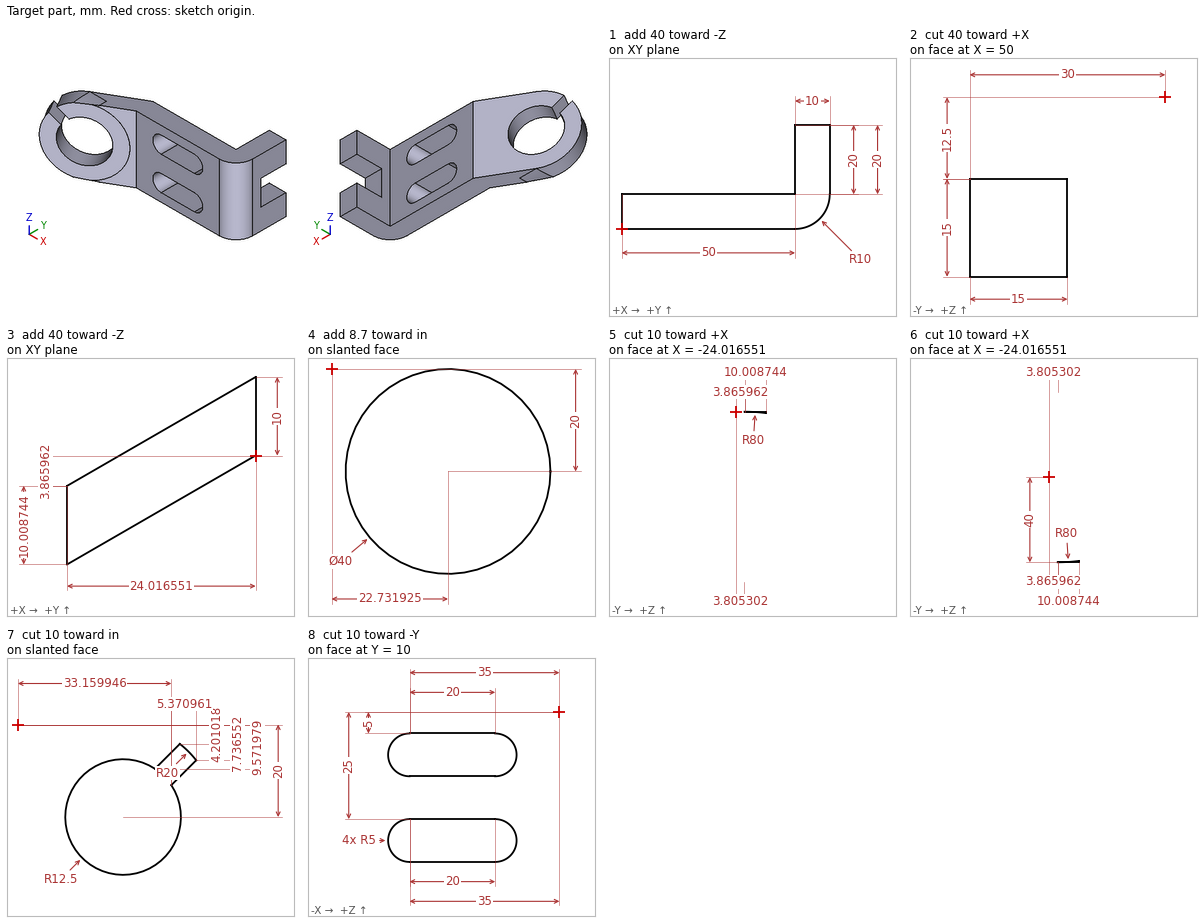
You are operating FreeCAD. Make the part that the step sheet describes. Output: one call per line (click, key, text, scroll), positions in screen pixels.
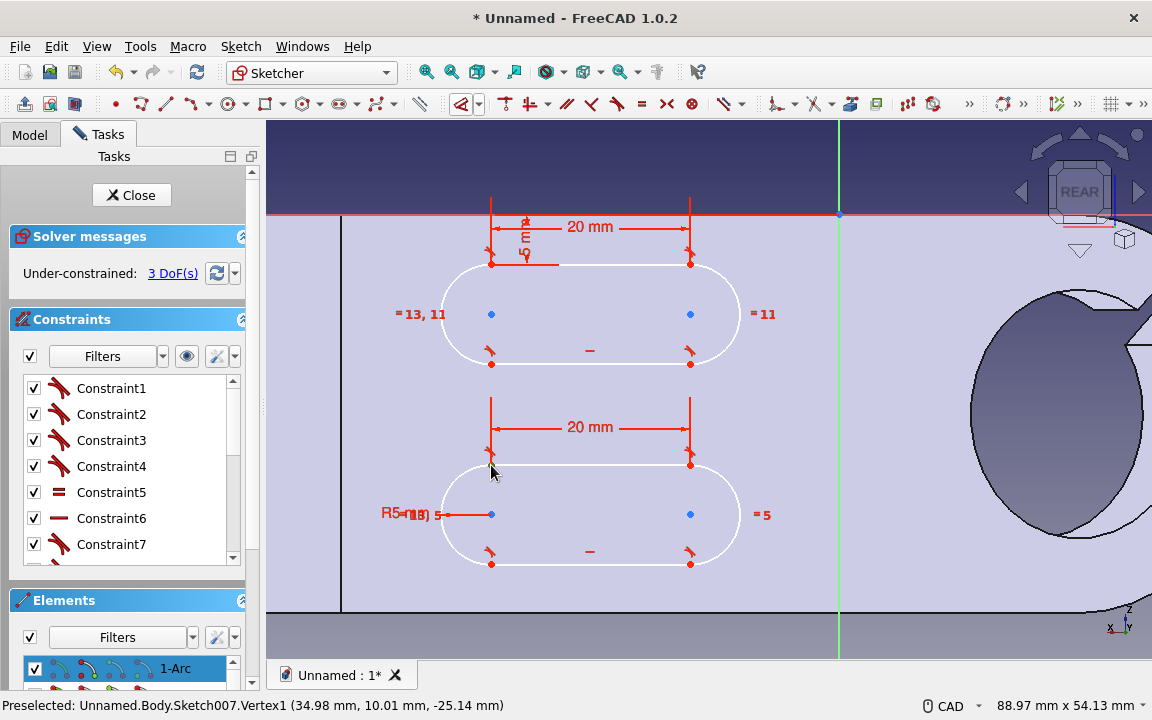
key(l)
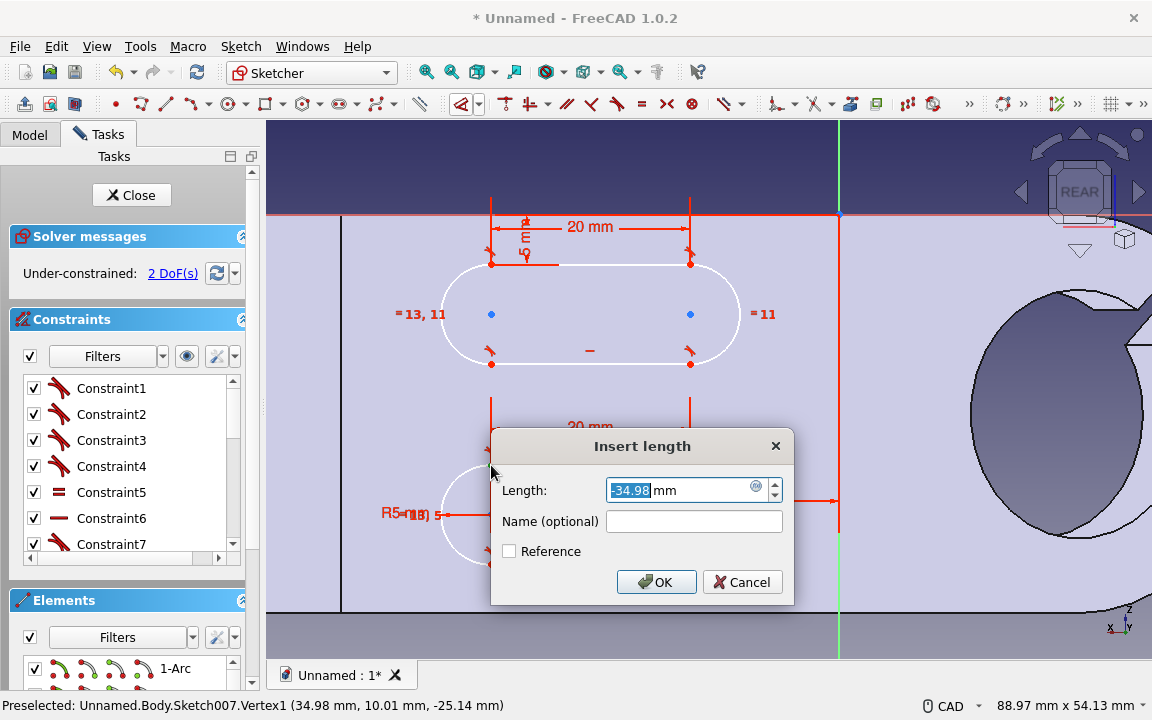
text(-35)
key(Return)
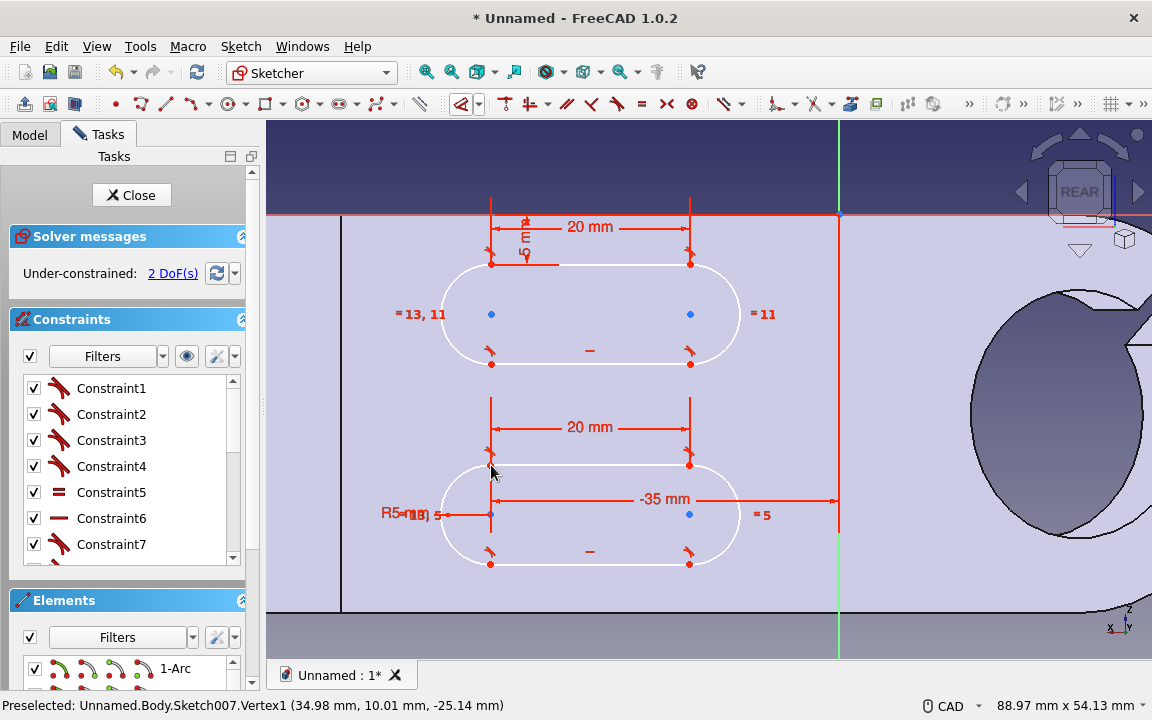
click(491, 465)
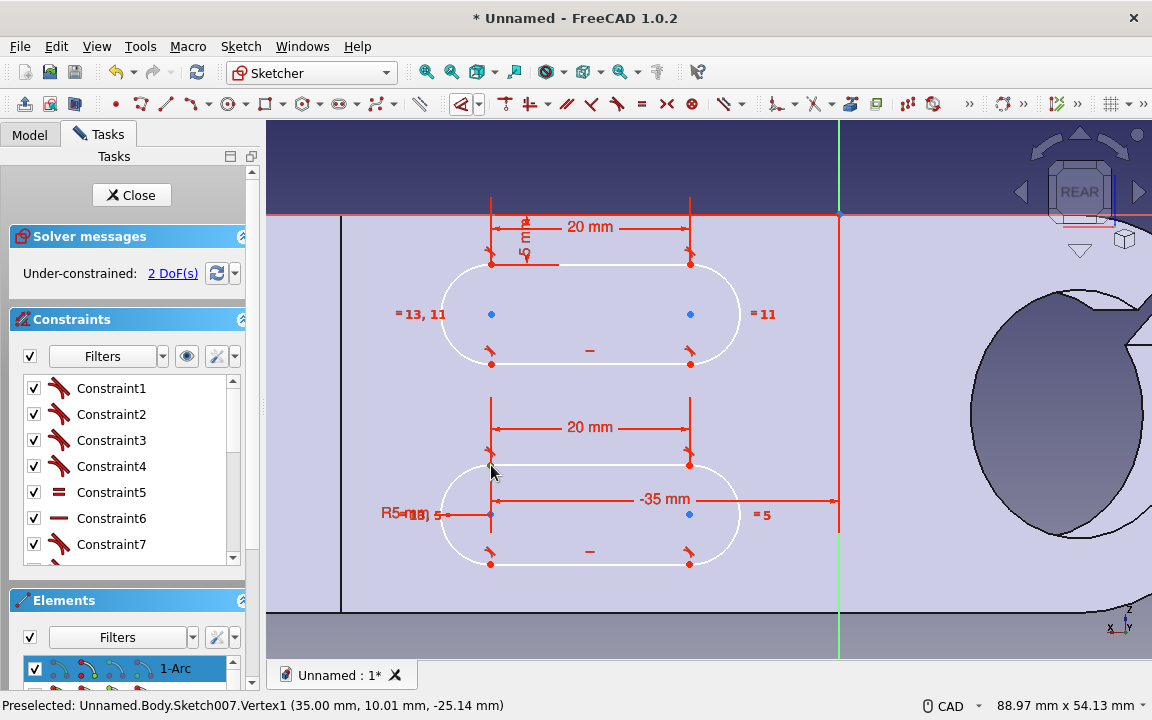
key(i)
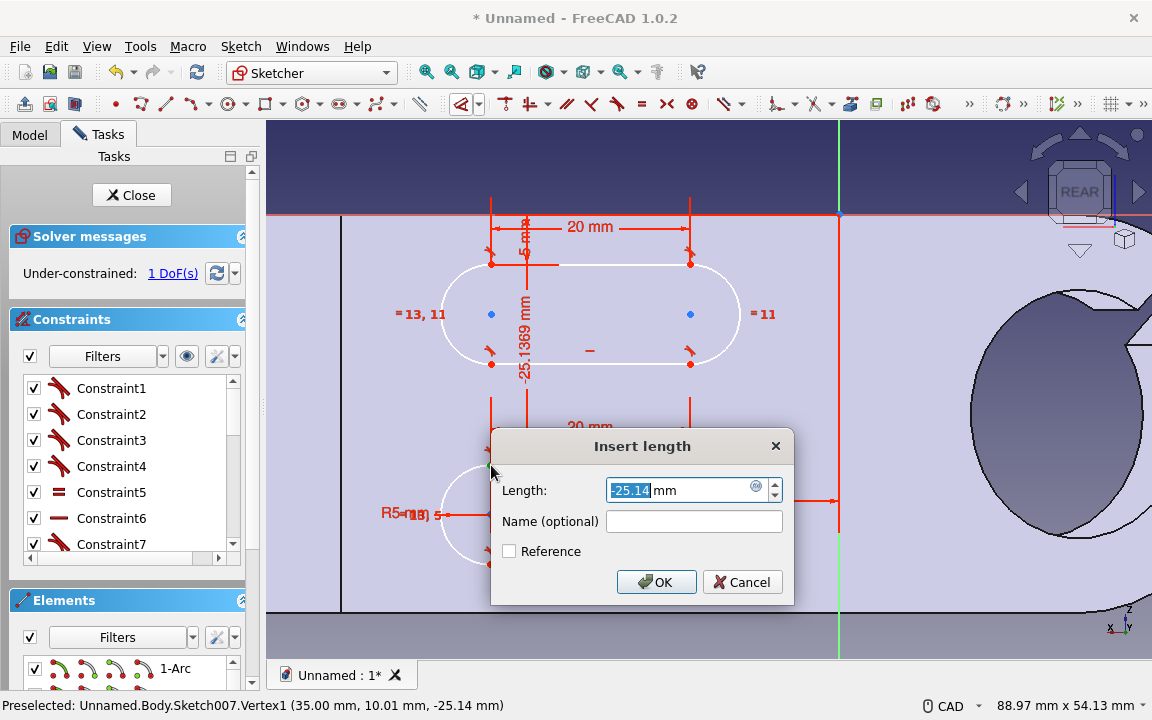
text(-25)
key(Return)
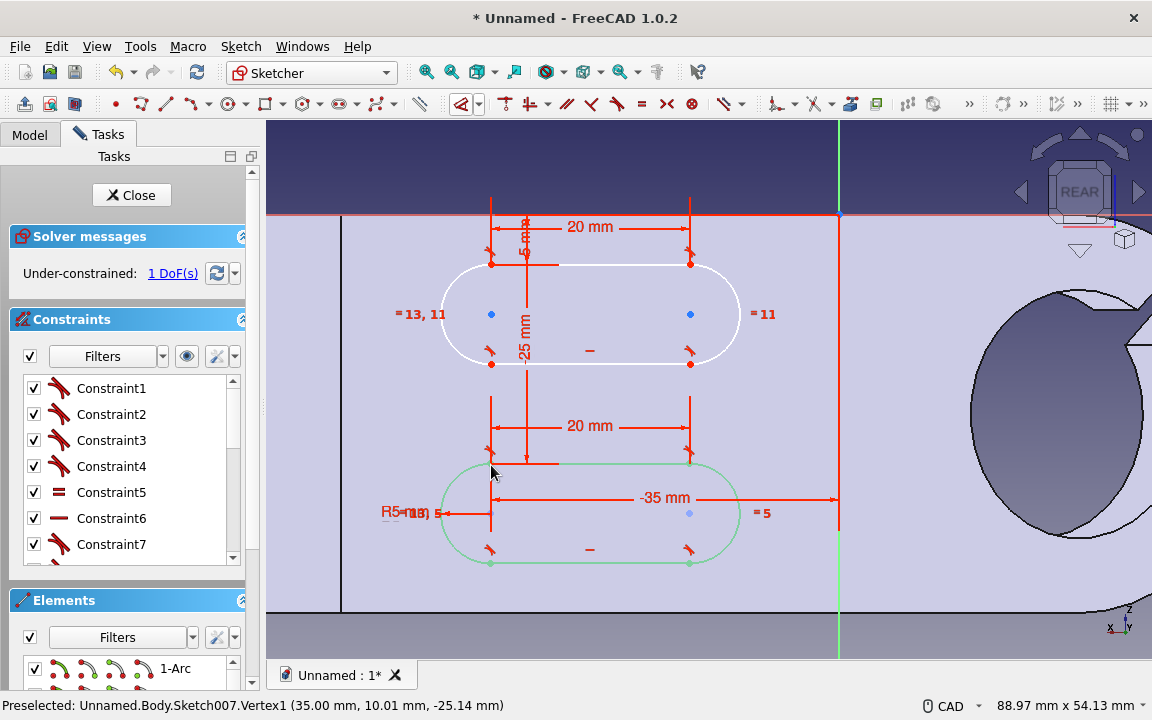
click(491, 265)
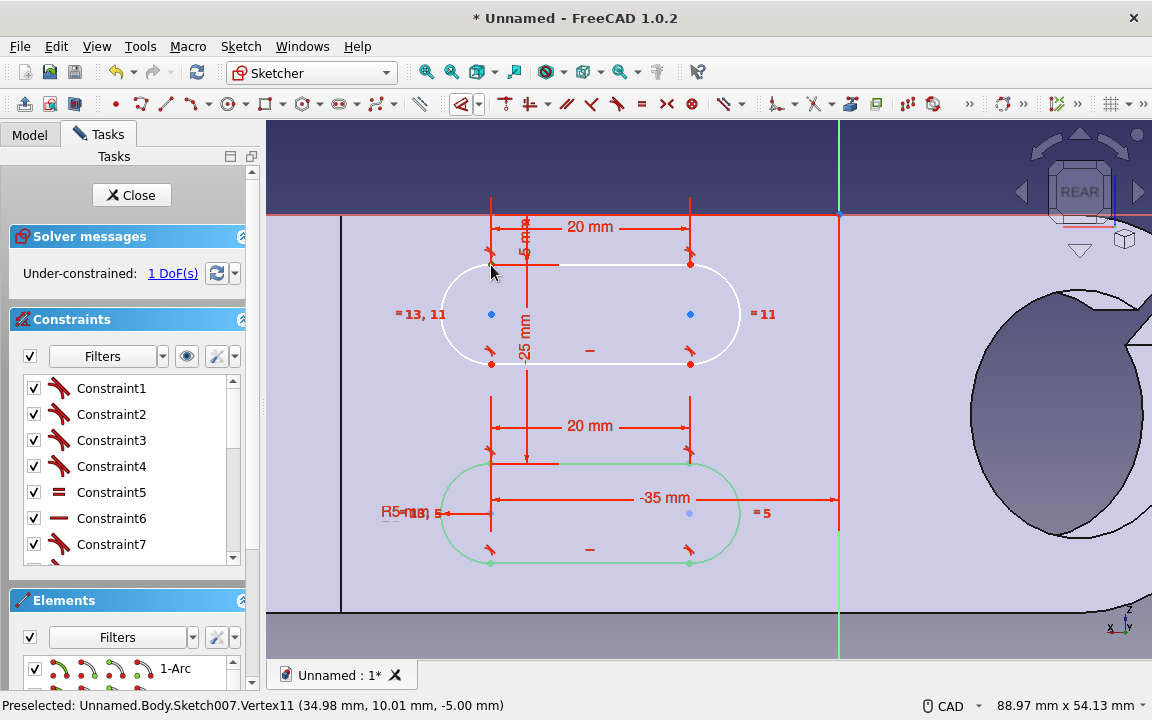
key(l)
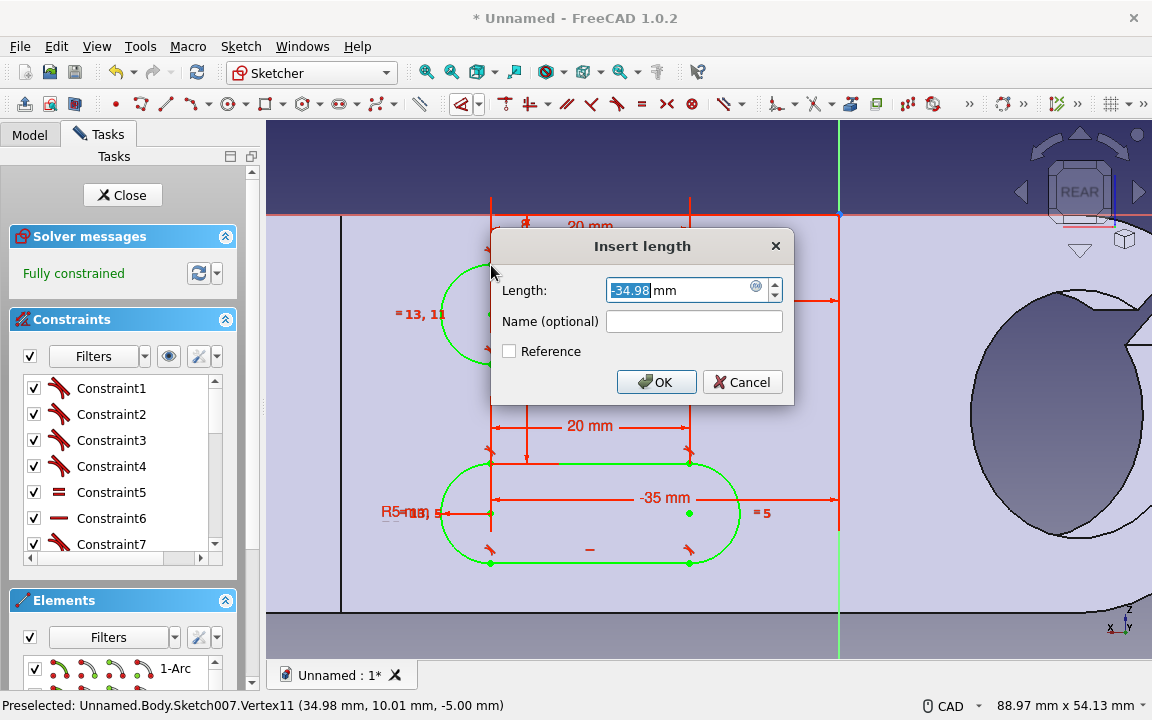
text(-35)
key(Return)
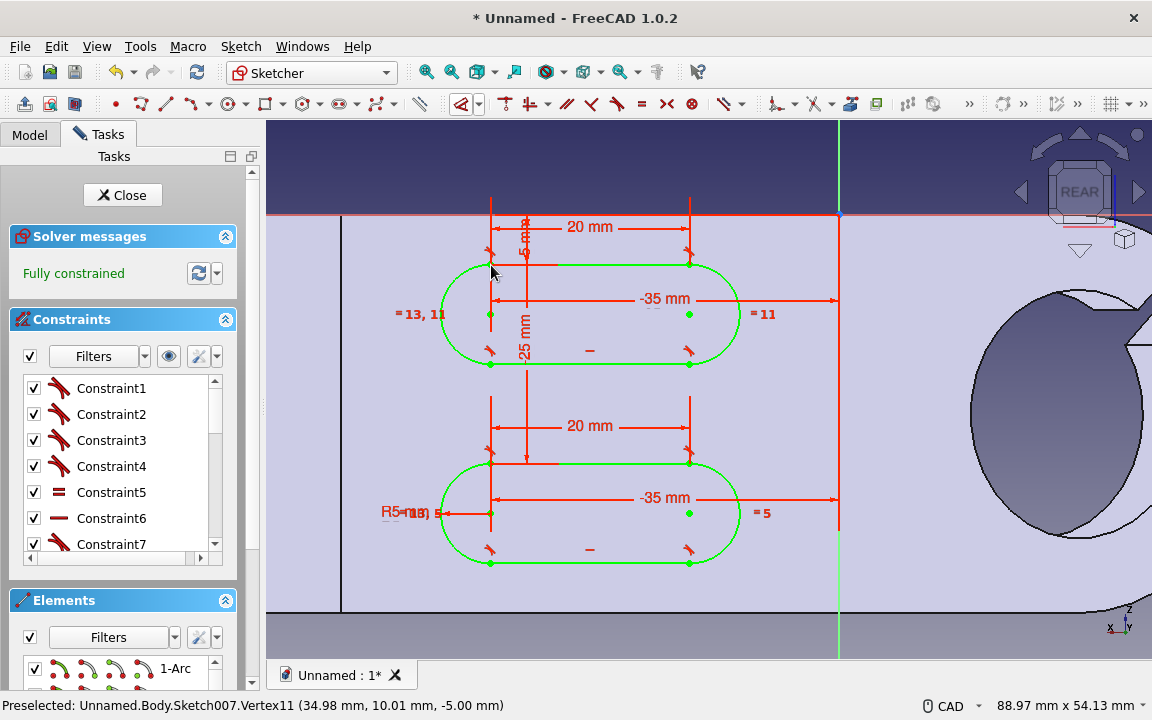
click(123, 195)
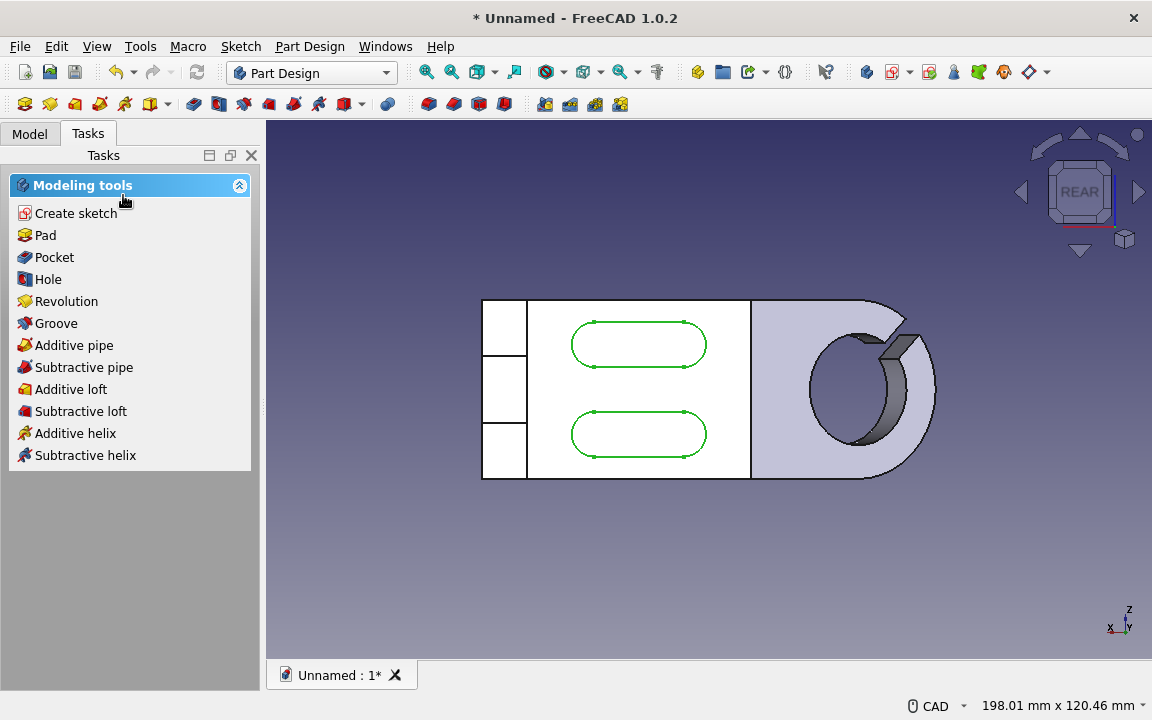
click(194, 104)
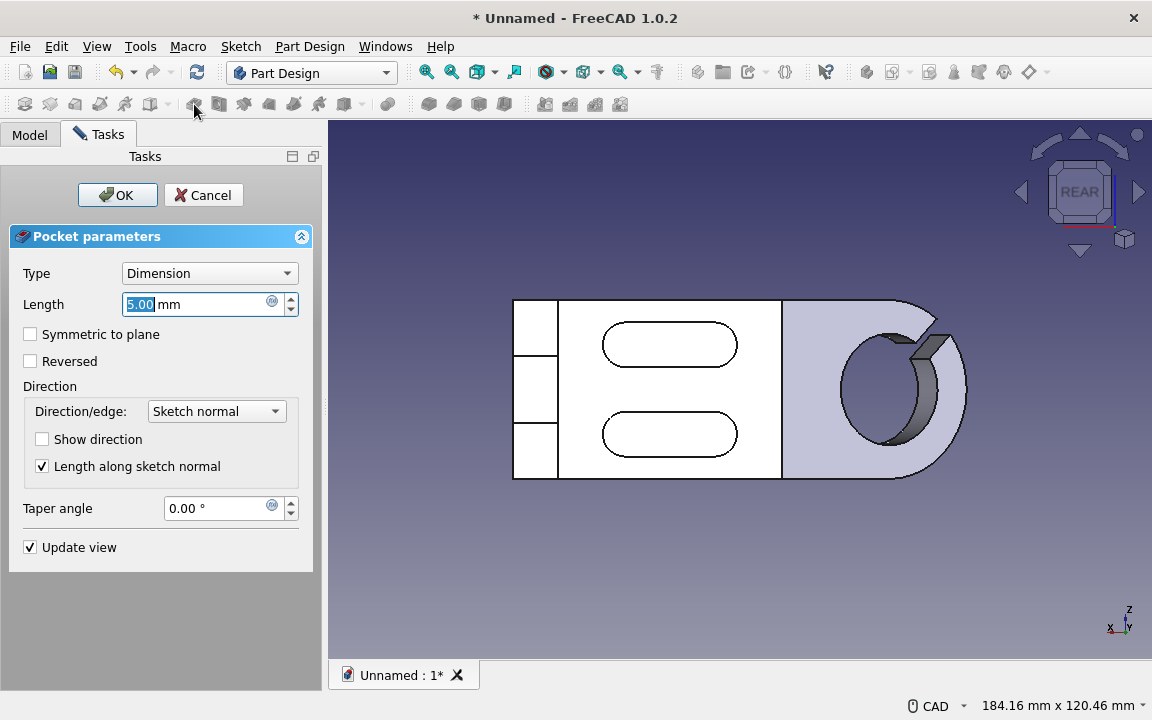
text(10)
key(Tab)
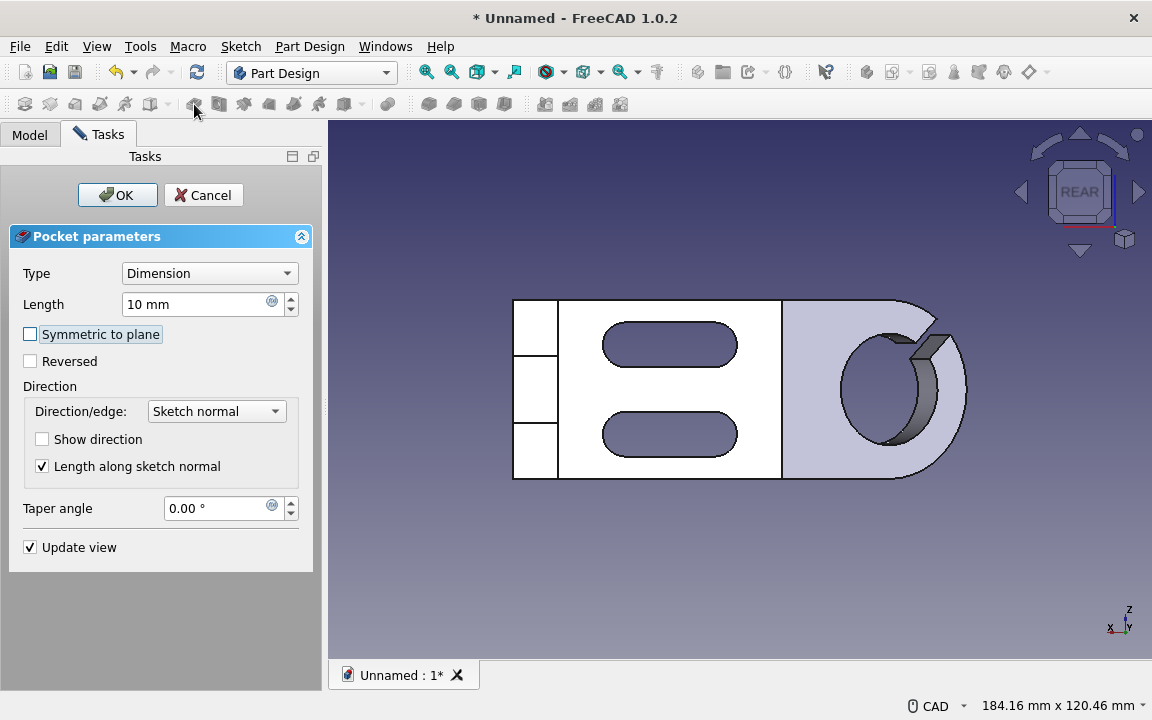
click(118, 195)